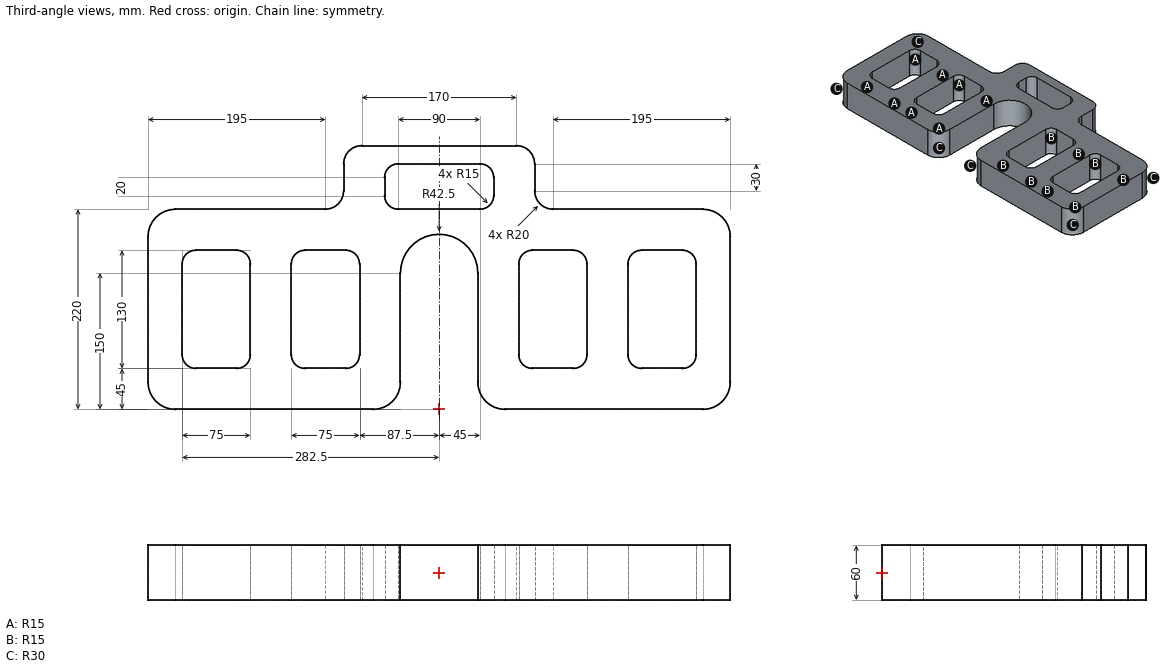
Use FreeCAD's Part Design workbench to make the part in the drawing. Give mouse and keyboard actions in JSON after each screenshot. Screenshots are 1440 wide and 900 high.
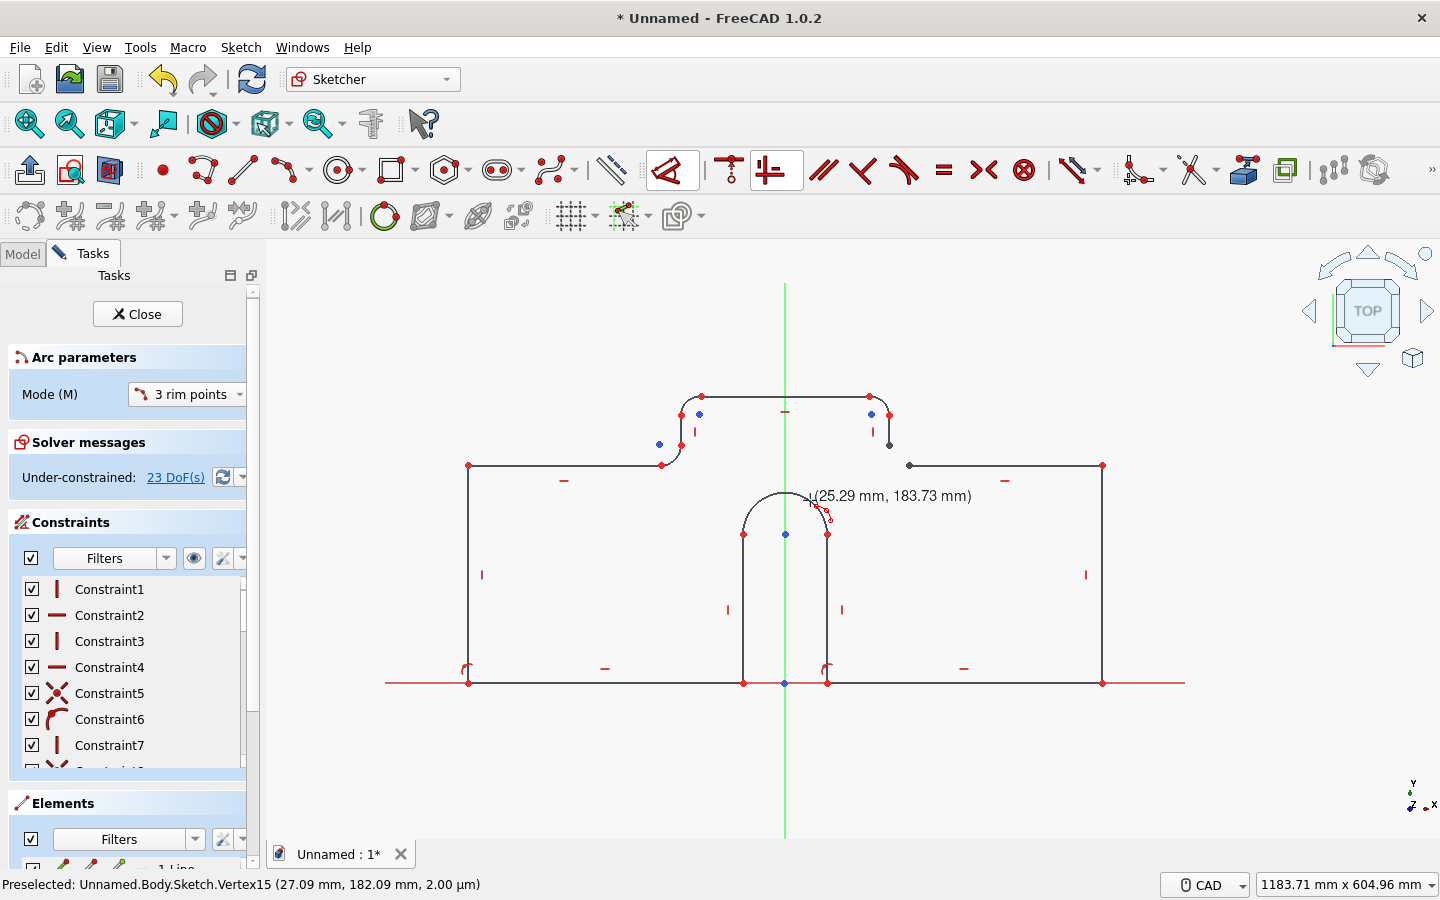
{"action": "left_click", "coordinate": [909, 466]}
{"action": "left_click", "coordinate": [889, 446]}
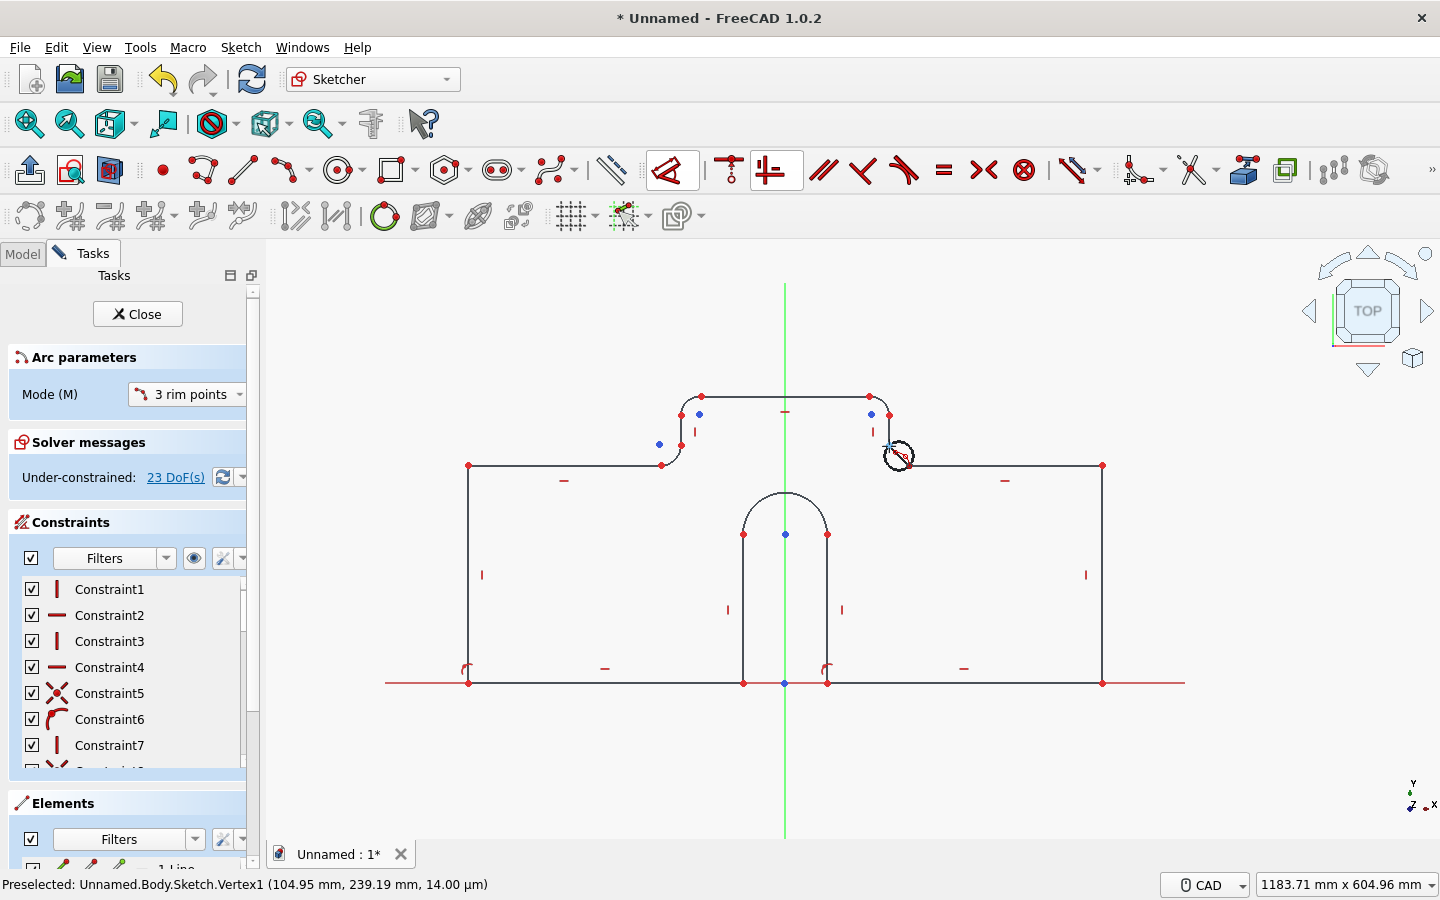
{"action": "scroll", "coordinate": [895, 459], "scroll_direction": "up", "scroll_amount": 6}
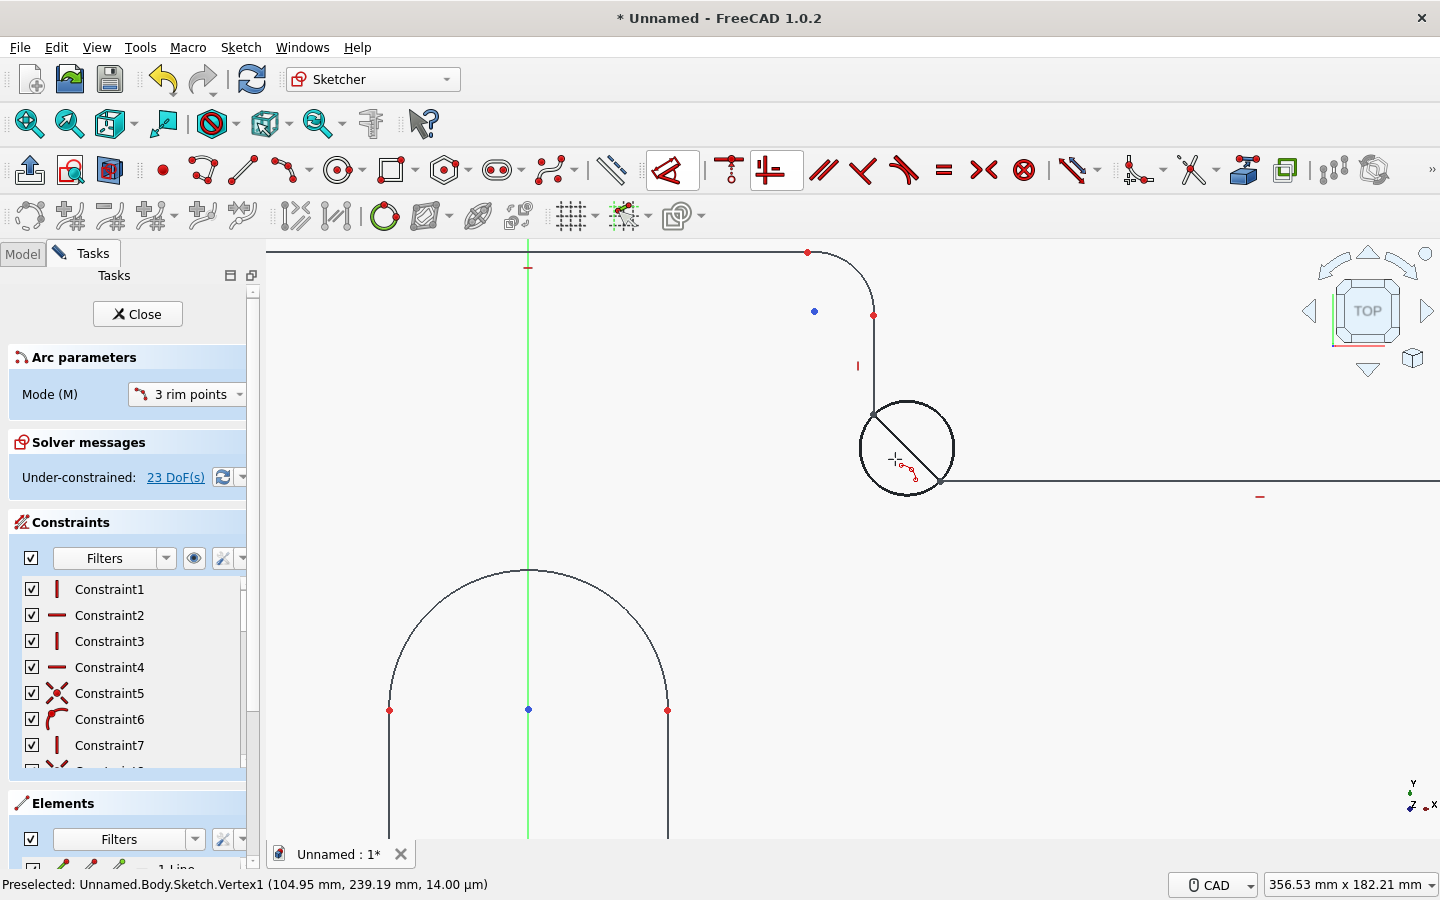
{"action": "left_click", "coordinate": [893, 459]}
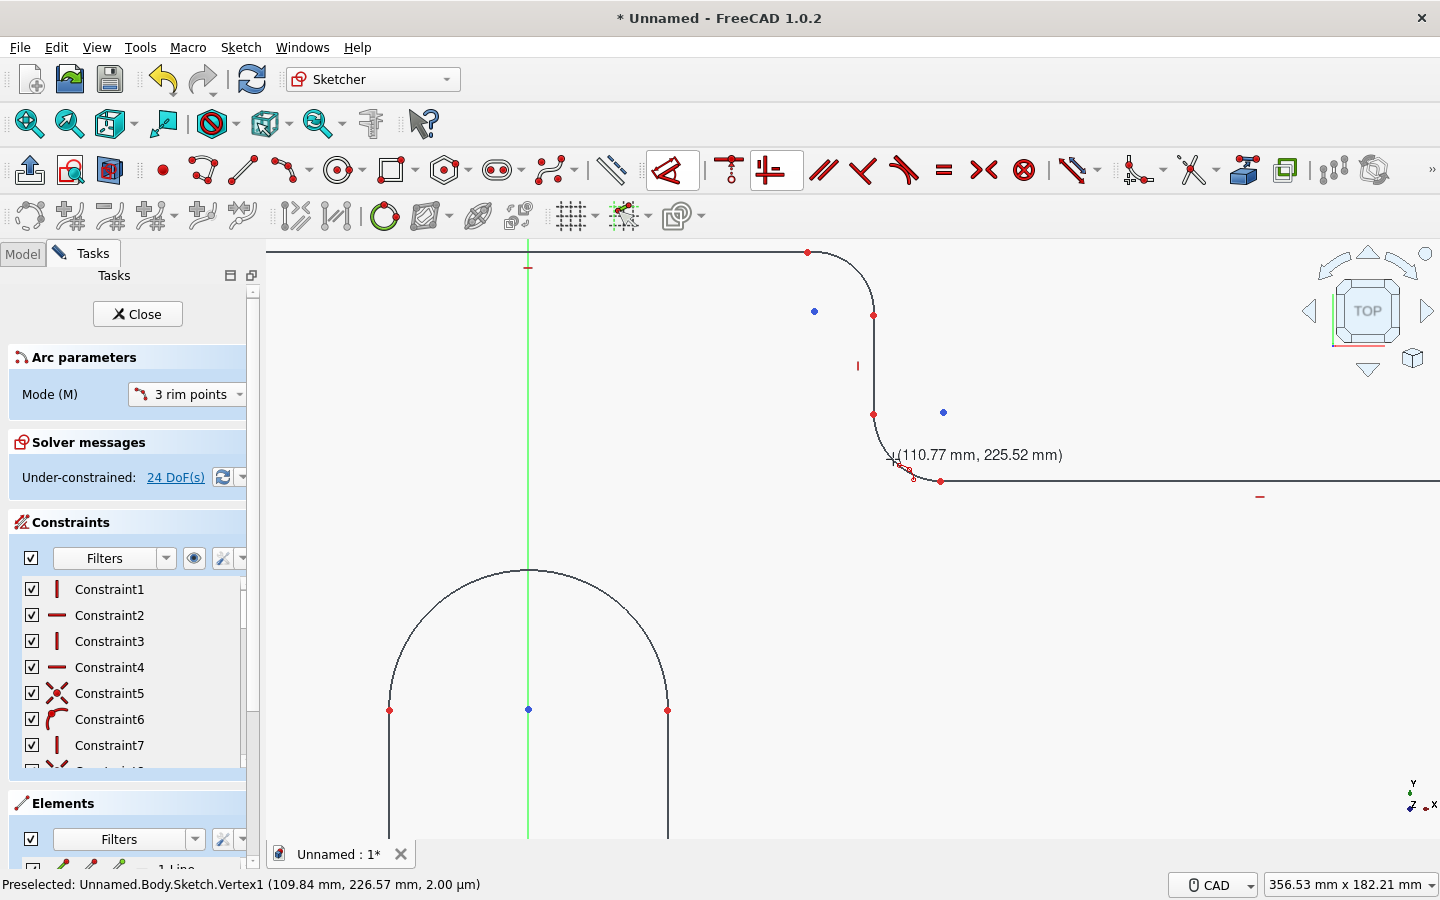
{"action": "left_click", "coordinate": [244, 170]}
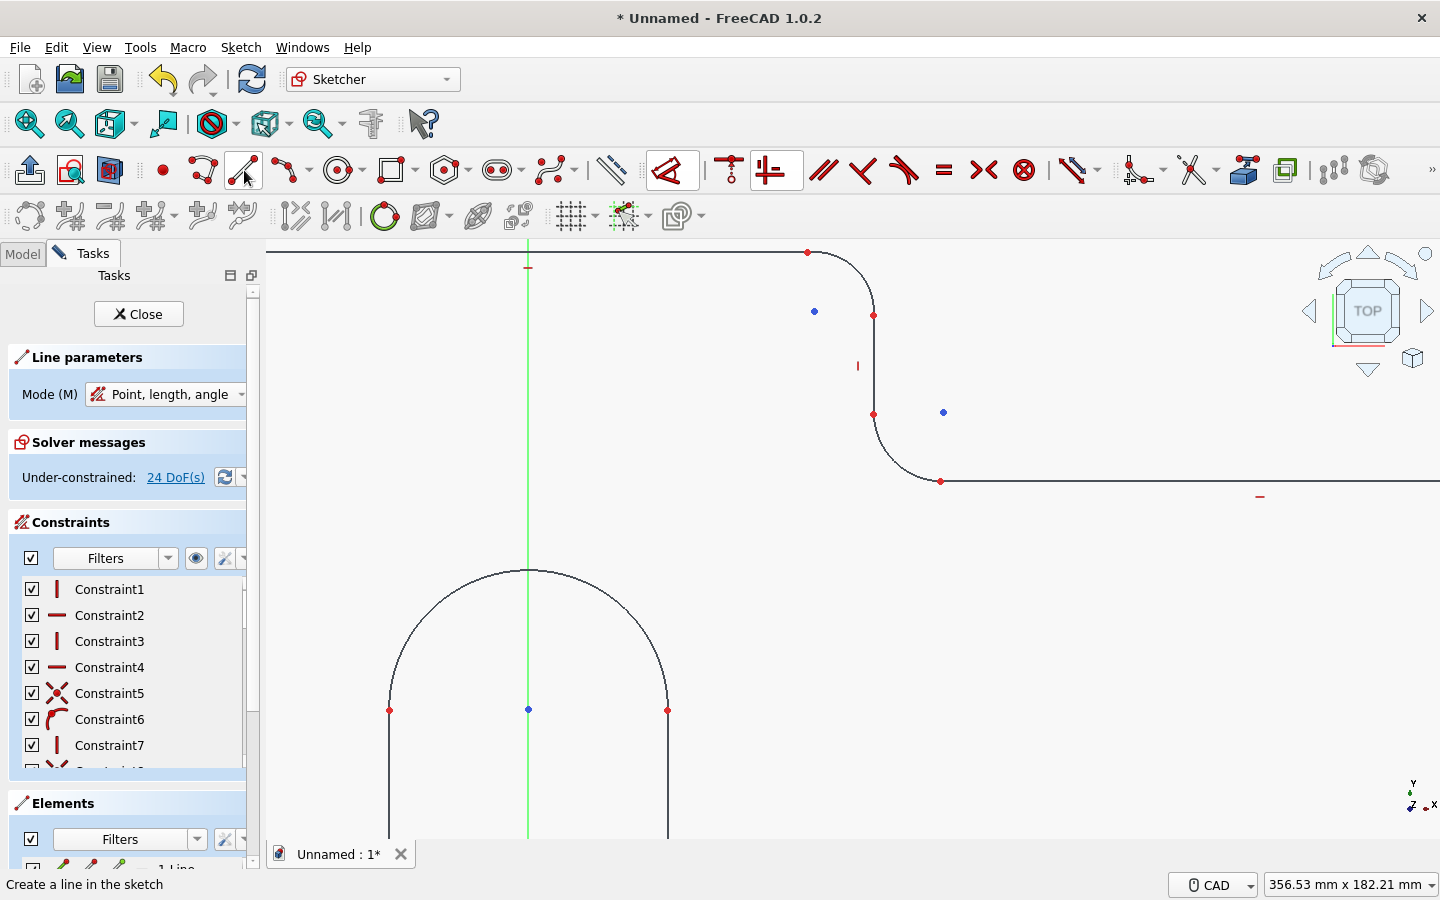
{"action": "left_click", "coordinate": [676, 478]}
{"action": "left_click", "coordinate": [380, 478]}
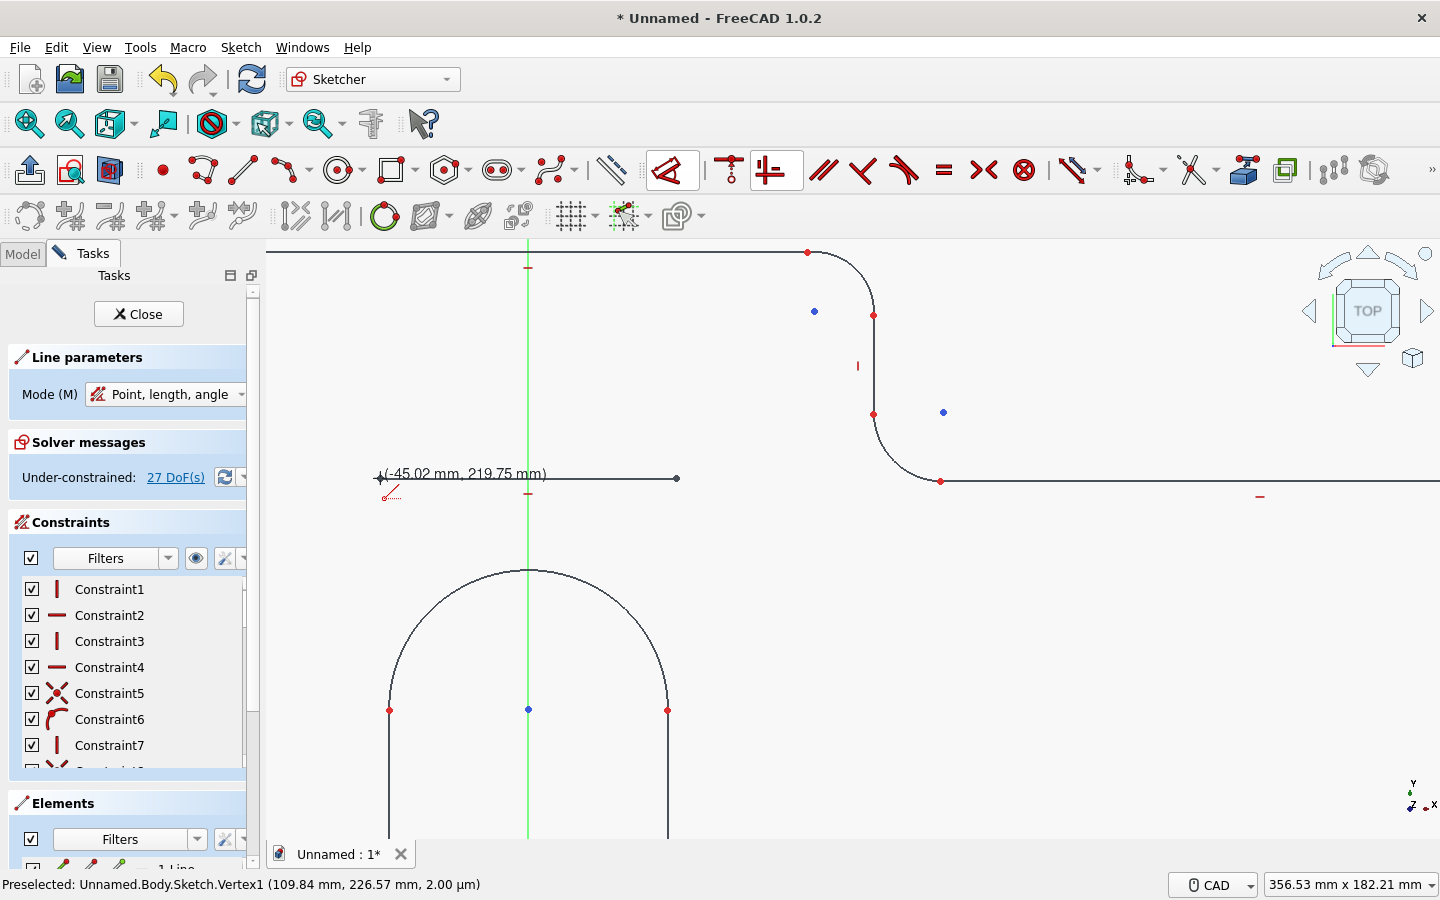
{"action": "left_click", "coordinate": [331, 429]}
{"action": "left_click", "coordinate": [331, 363]}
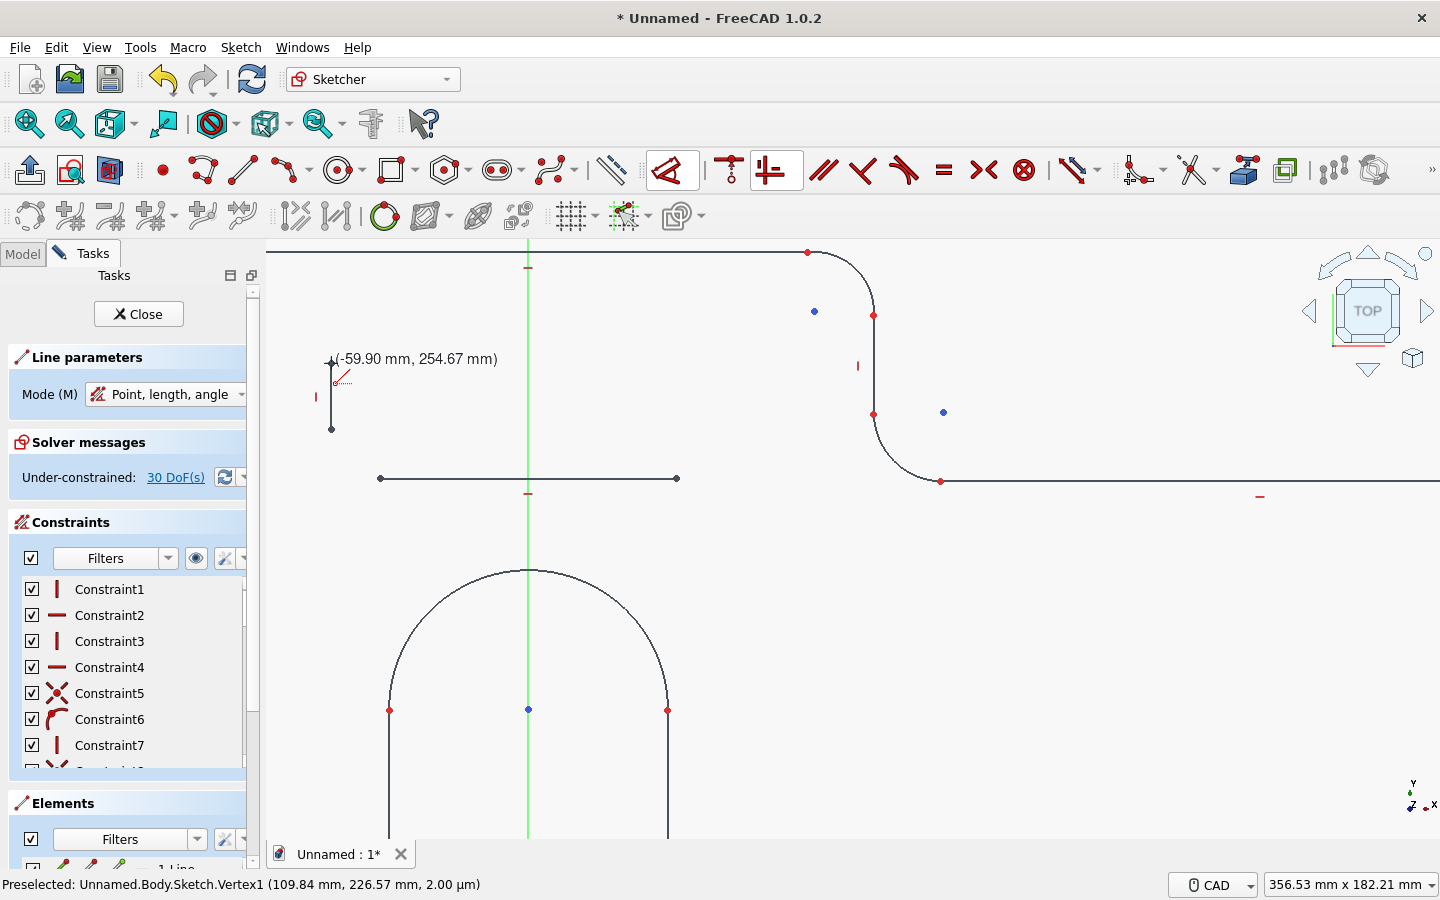
{"action": "left_click", "coordinate": [380, 314]}
{"action": "left_click", "coordinate": [676, 314]}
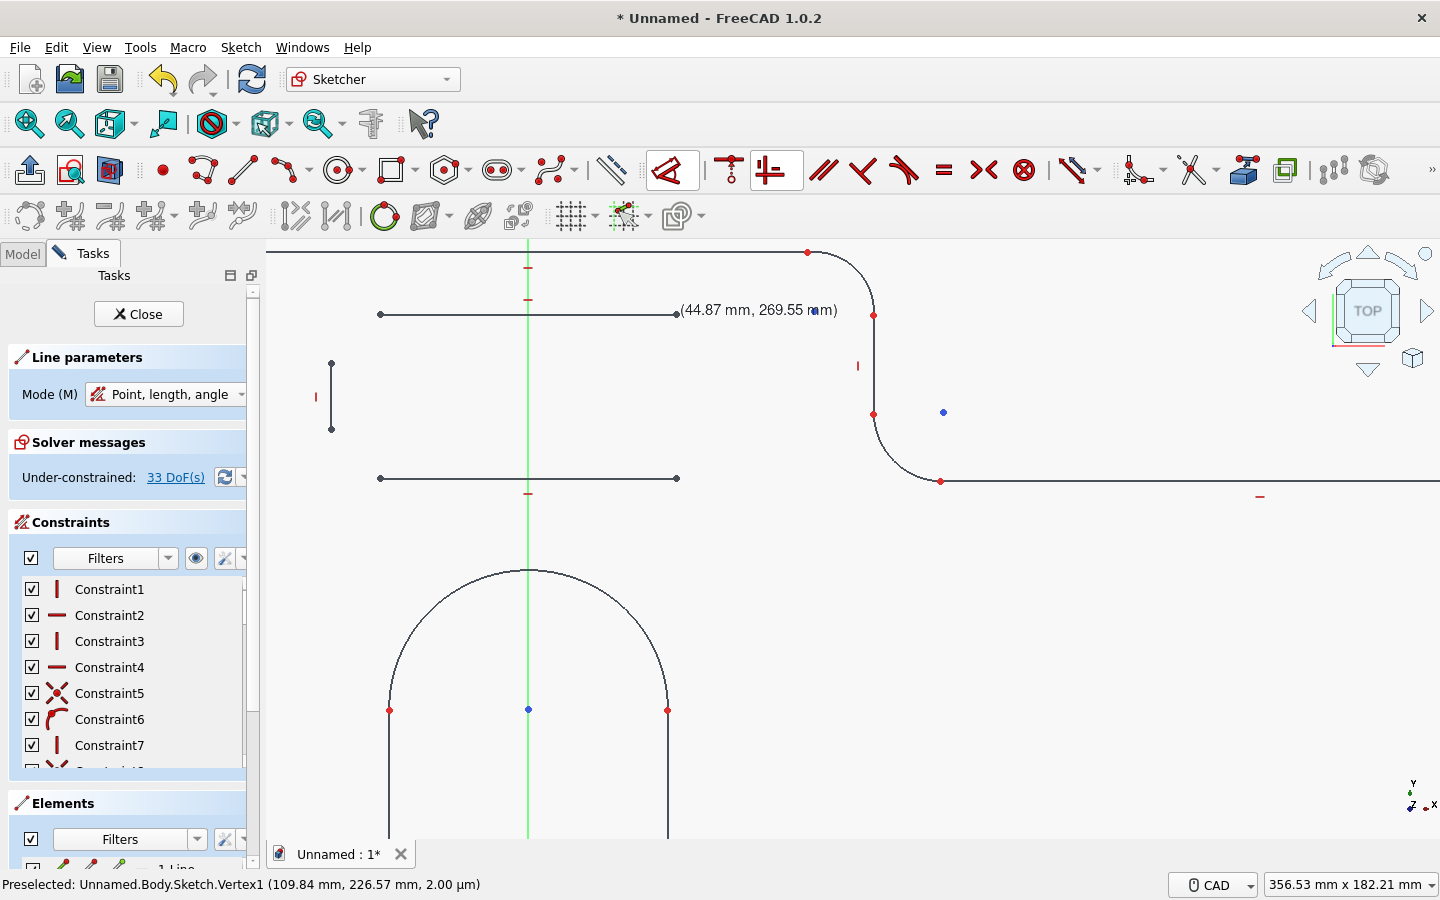
{"action": "left_click", "coordinate": [726, 363]}
{"action": "left_click", "coordinate": [726, 429]}